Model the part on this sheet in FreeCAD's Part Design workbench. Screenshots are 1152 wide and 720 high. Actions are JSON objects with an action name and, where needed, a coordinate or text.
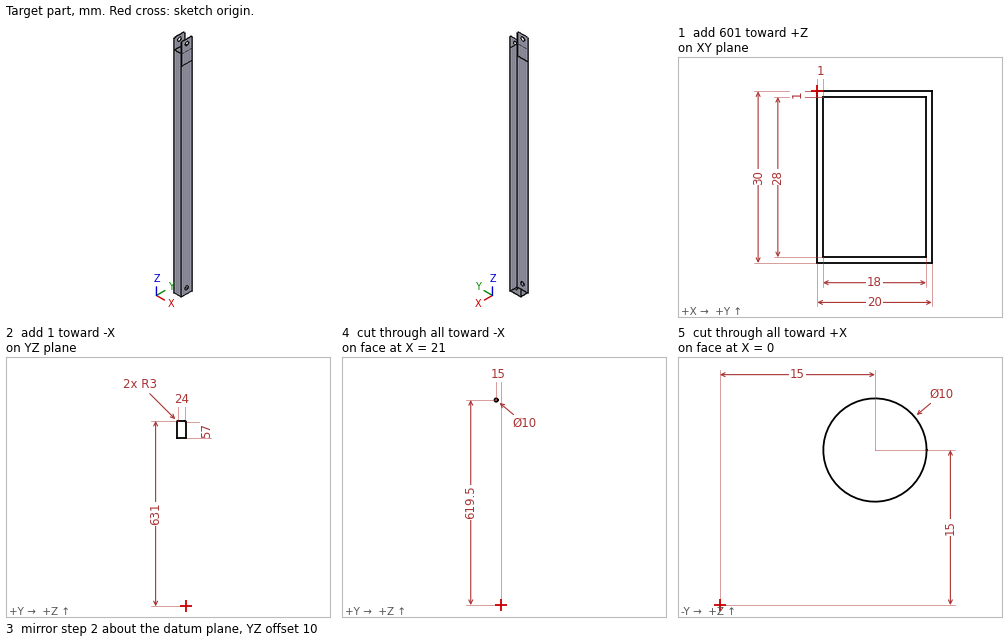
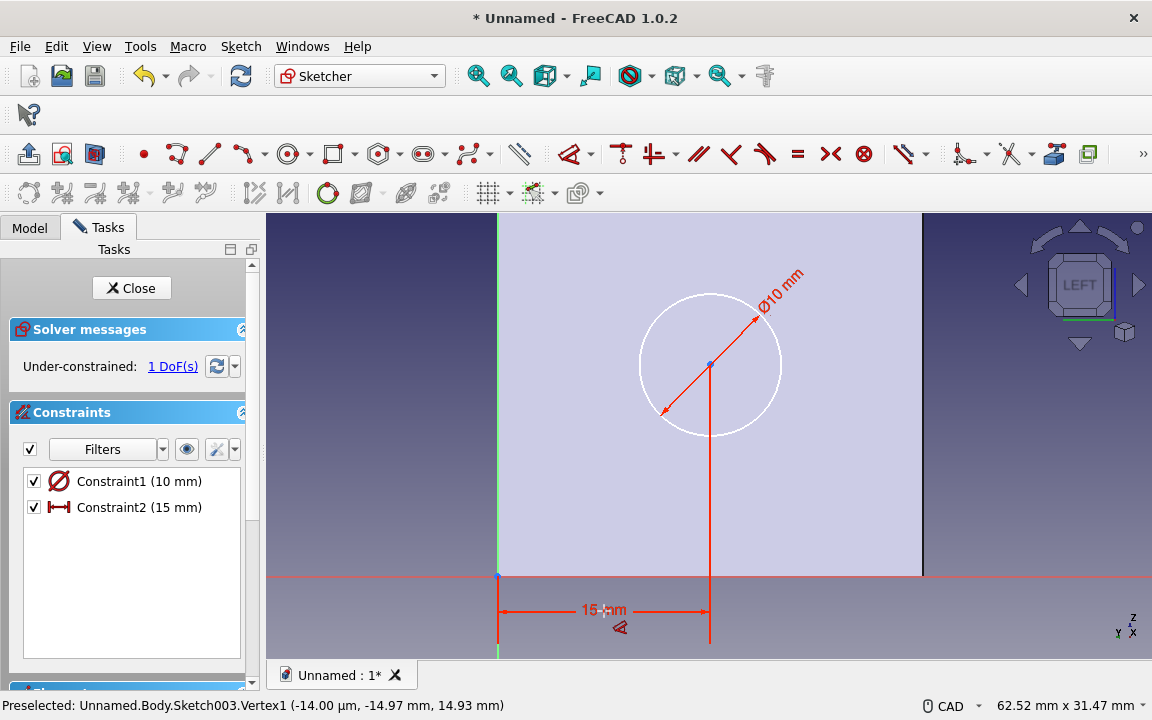
{"action": "left_click", "coordinate": [710, 365]}
{"action": "left_click", "coordinate": [464, 471]}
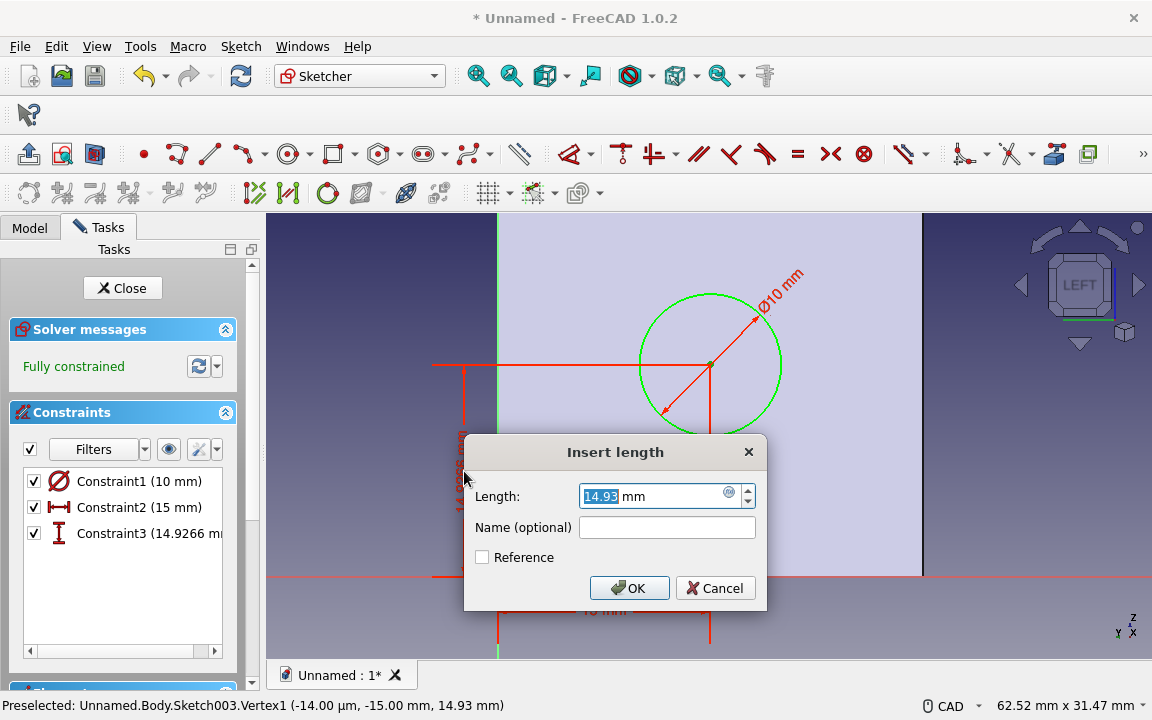
{"action": "type", "text": "15"}
{"action": "key", "text": "Return"}
{"action": "key", "text": "Escape"}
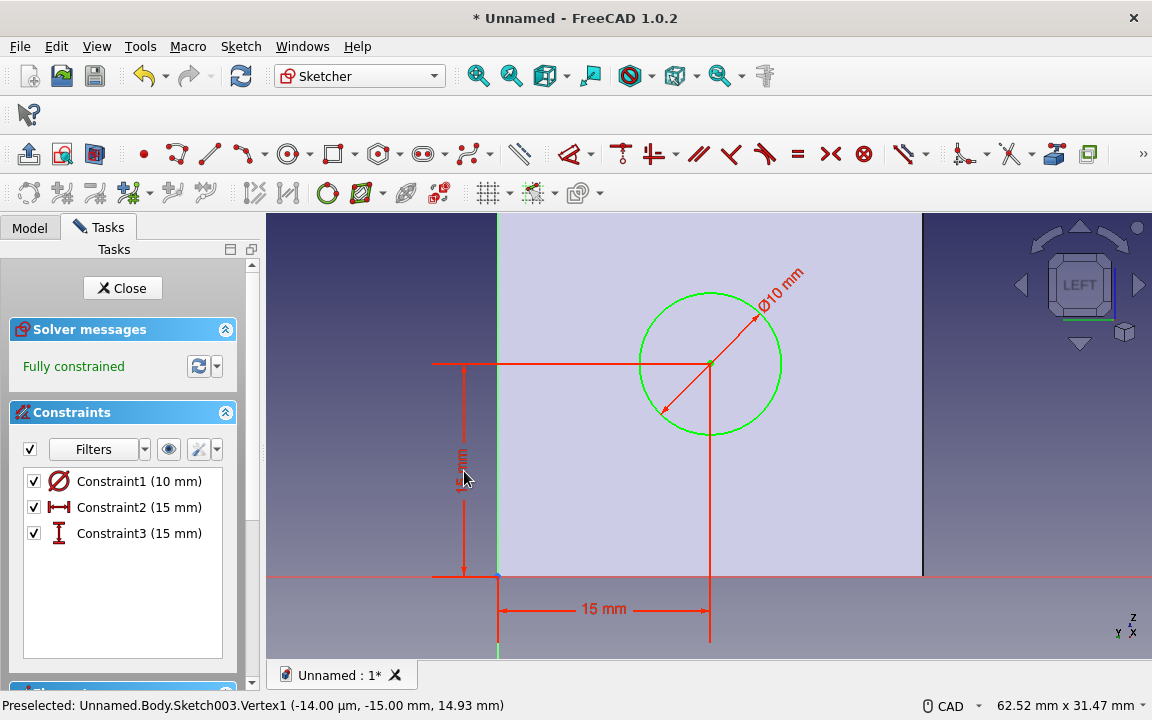
{"action": "left_click", "coordinate": [123, 288]}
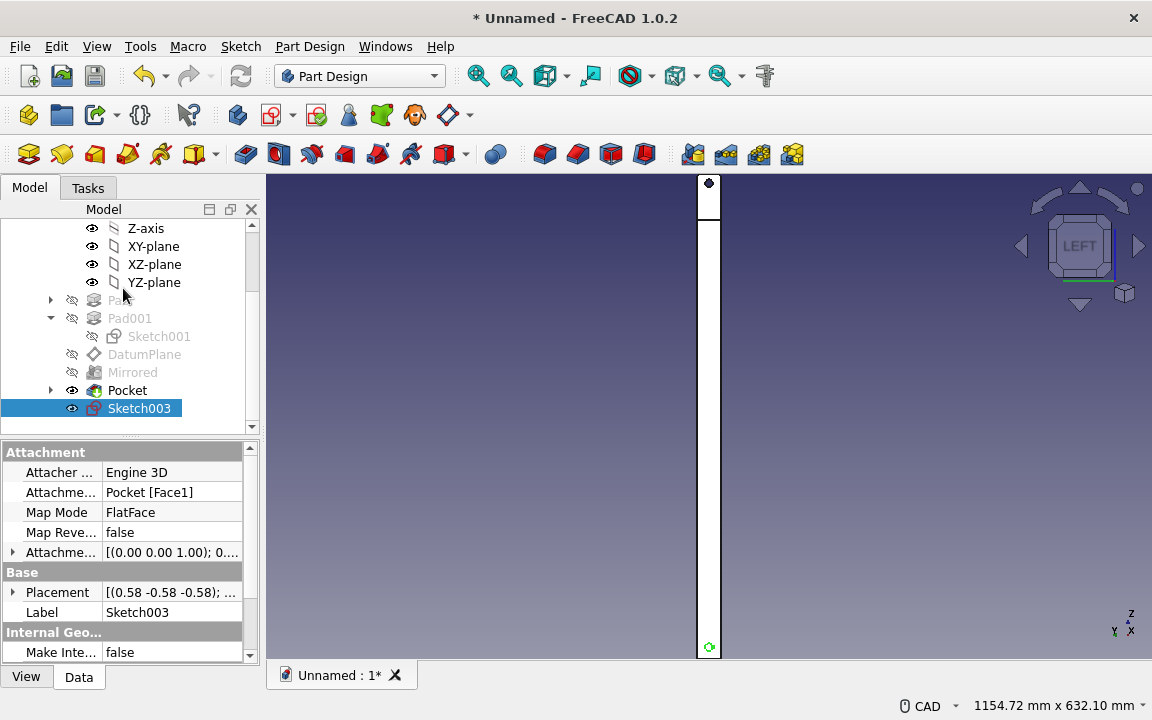
{"action": "left_click", "coordinate": [246, 154]}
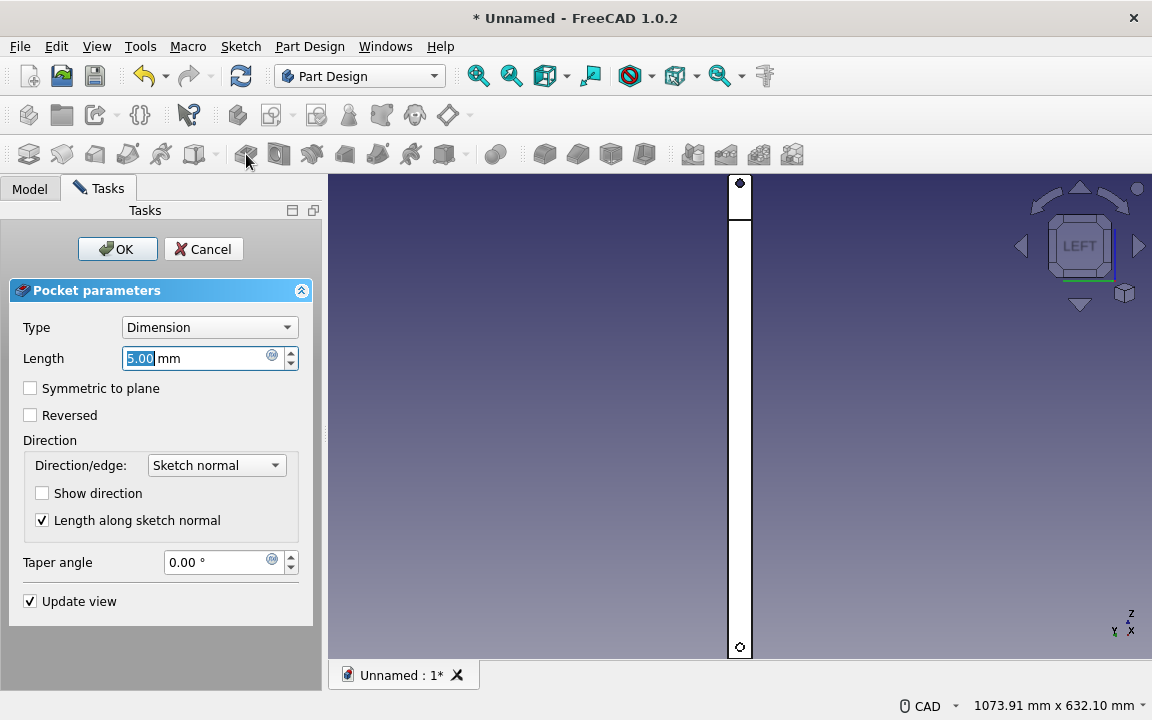
{"action": "left_click", "coordinate": [210, 328]}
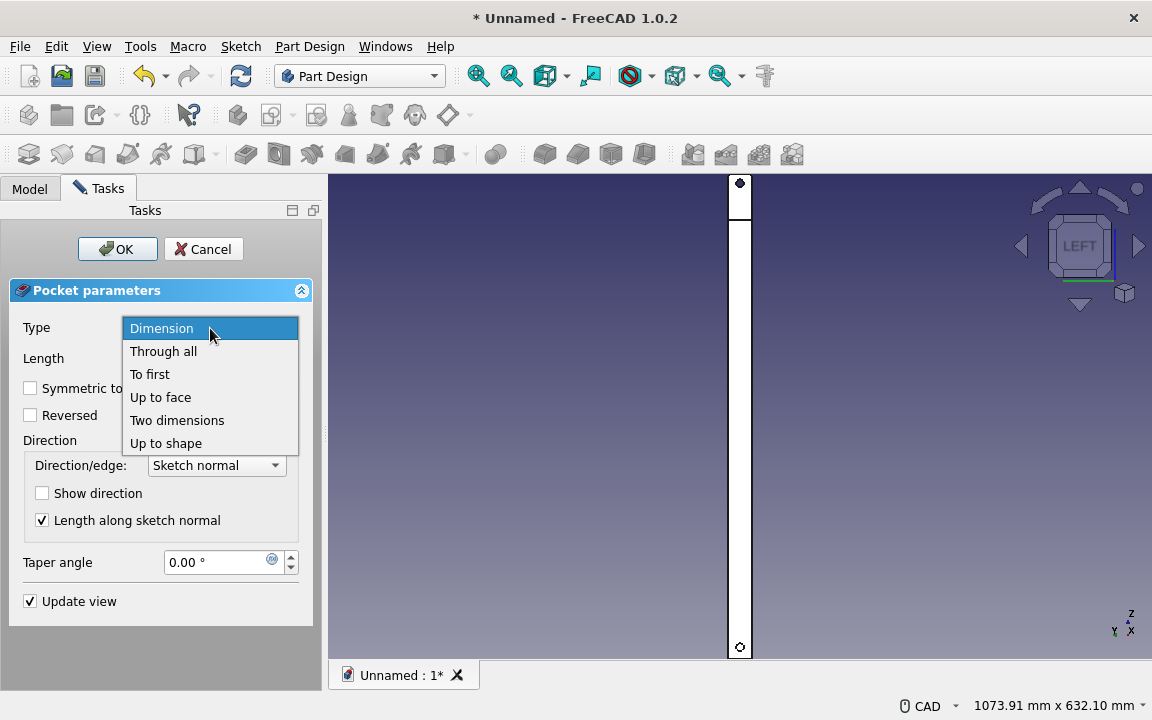
{"action": "left_click", "coordinate": [208, 352]}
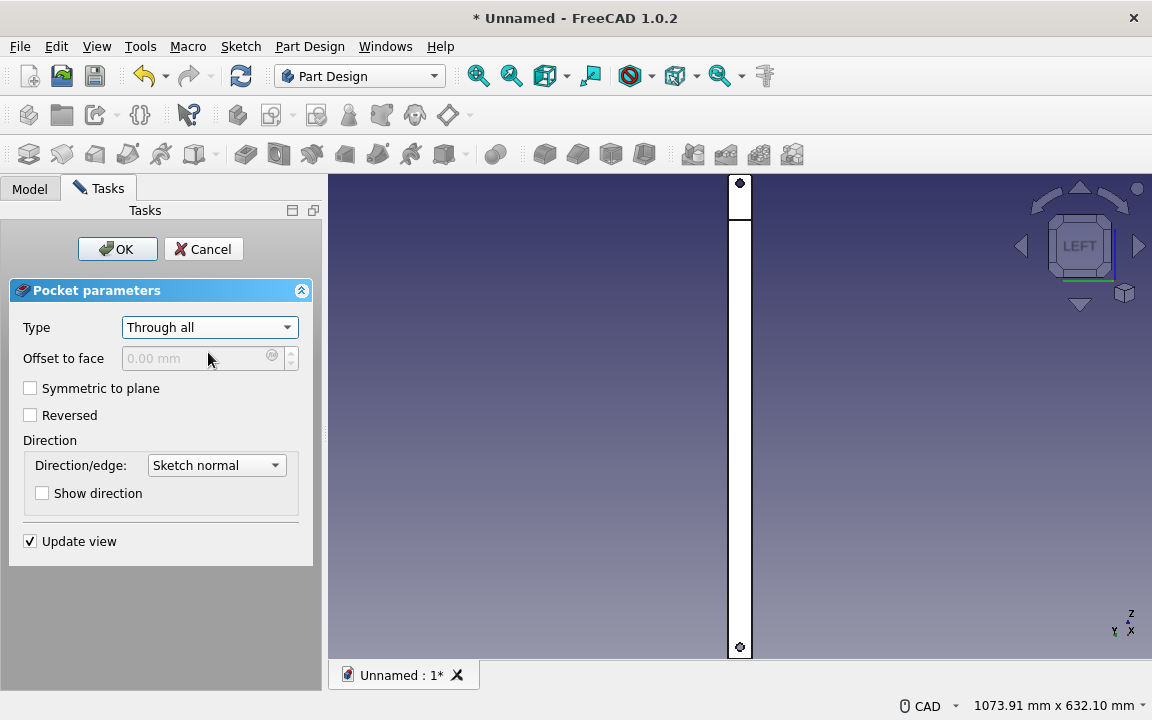
{"action": "left_click", "coordinate": [118, 249]}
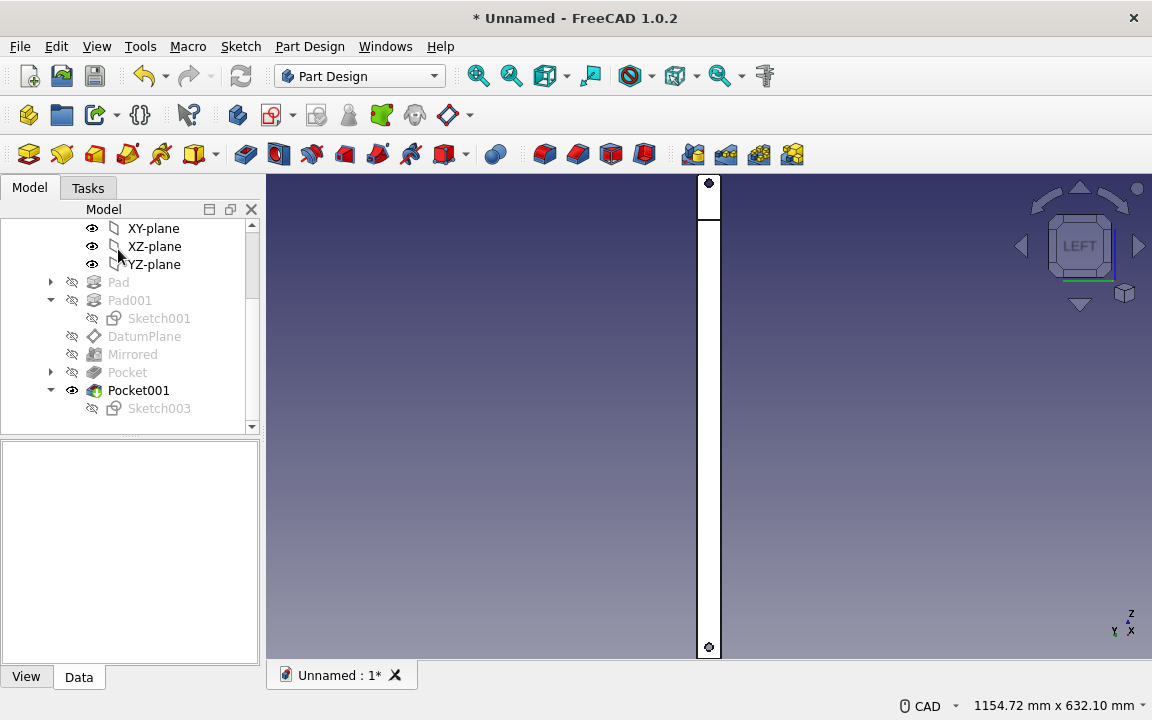
{"action": "key", "text": "0"}